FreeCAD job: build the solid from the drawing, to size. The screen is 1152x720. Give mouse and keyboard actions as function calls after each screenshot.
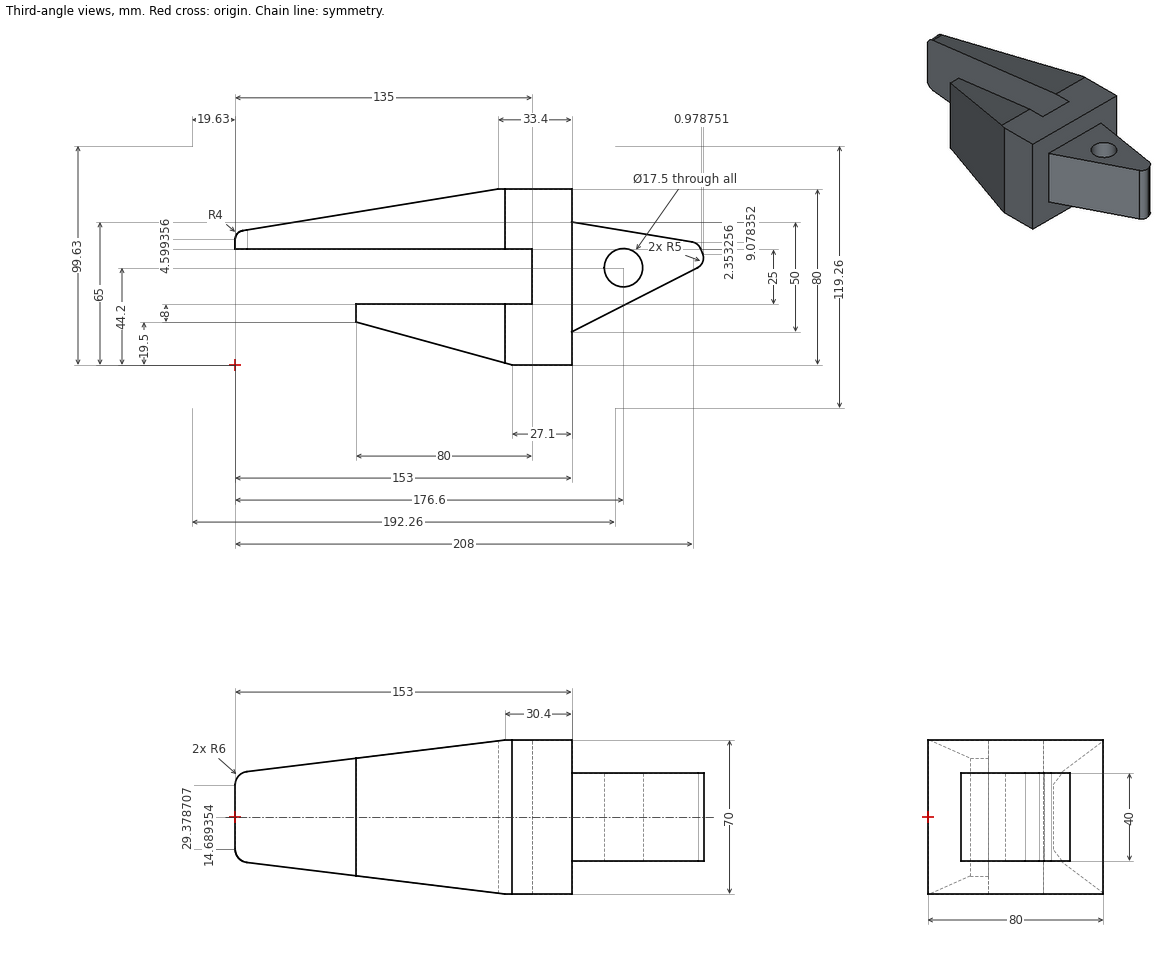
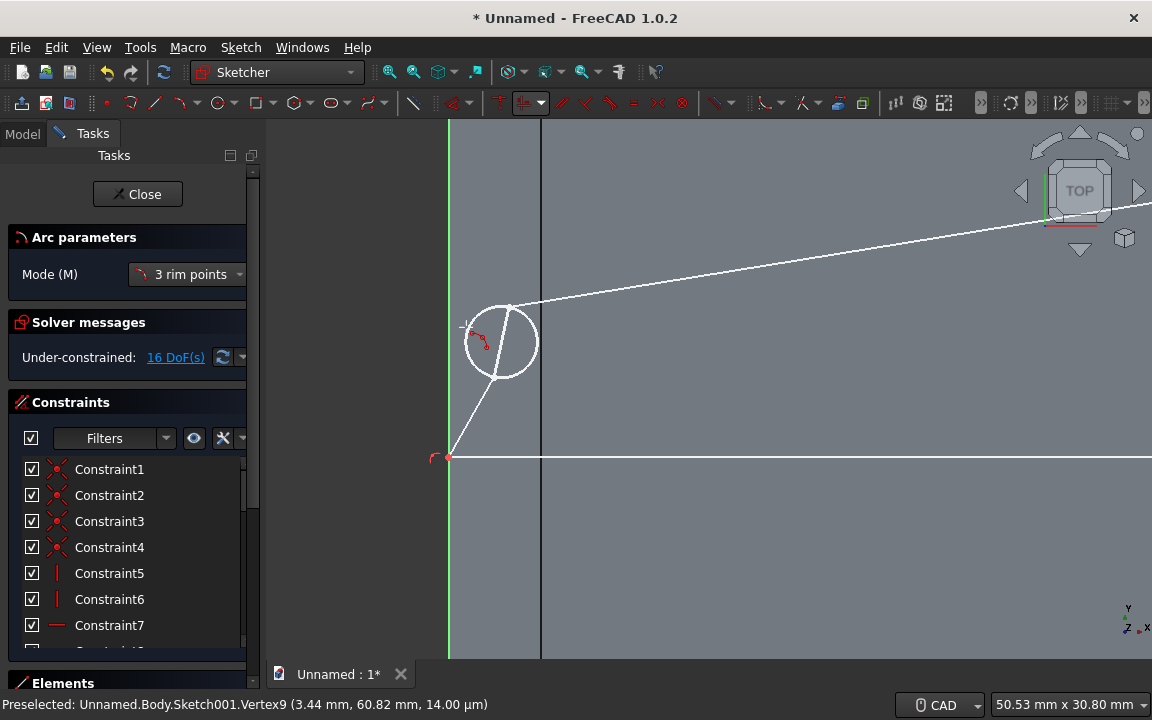
click(465, 327)
key(Escape)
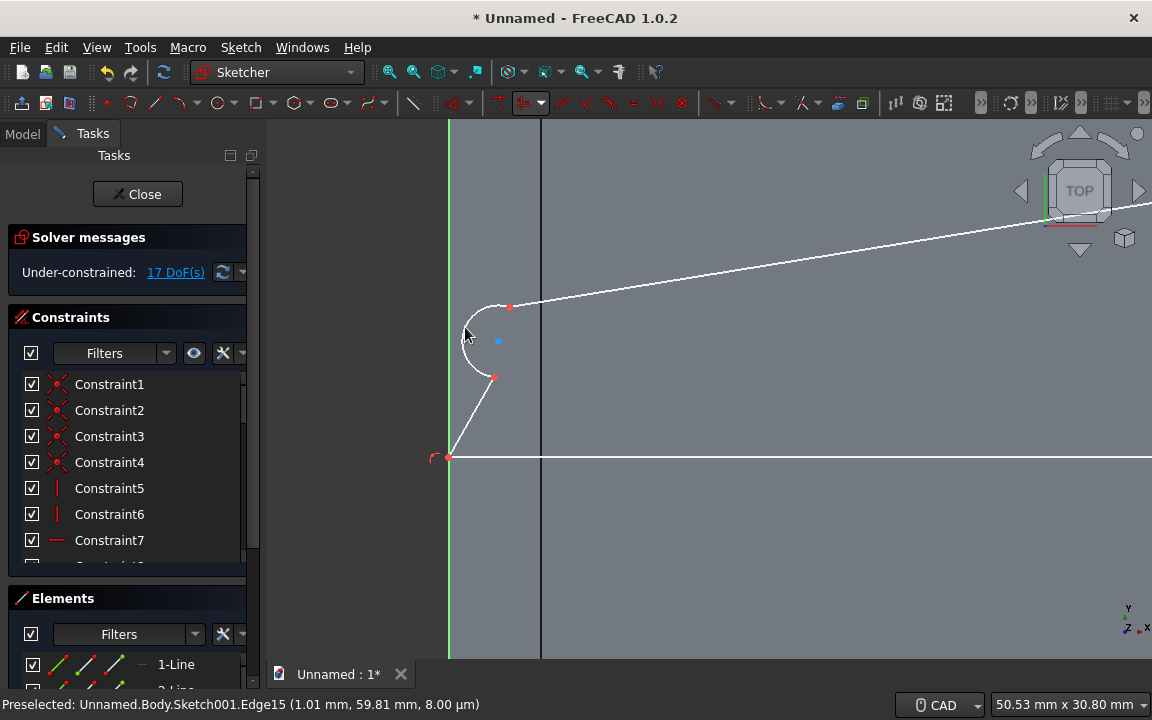
scroll(461, 345, down, 10)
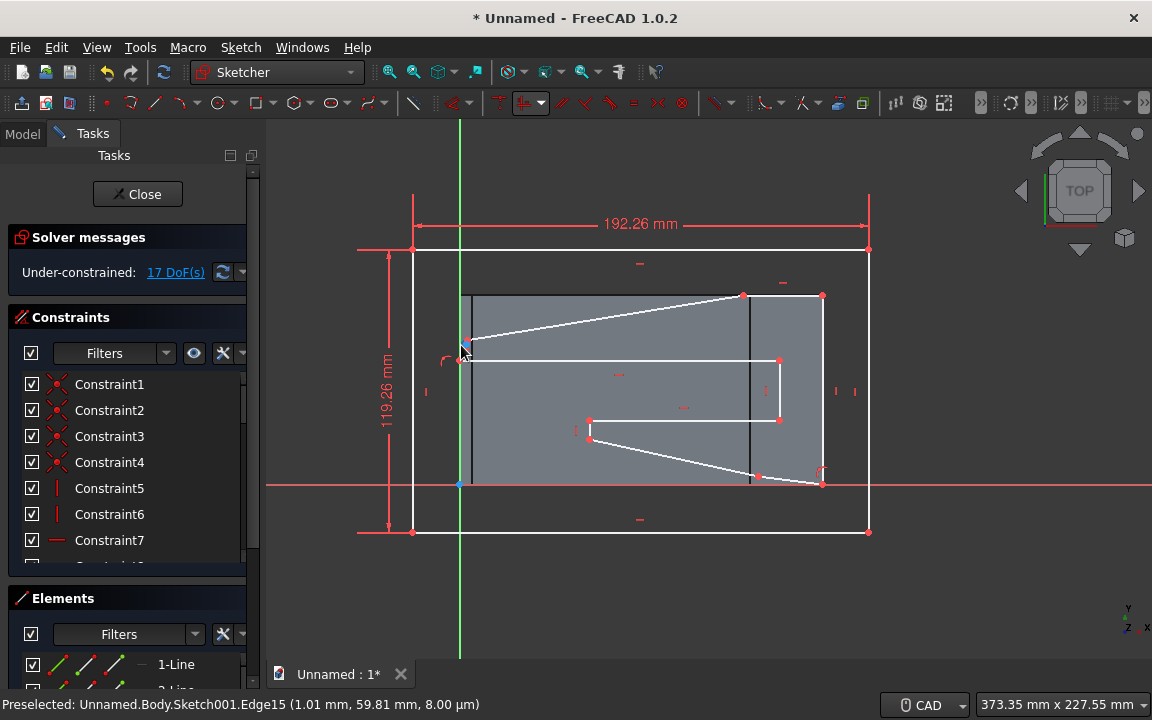
click(523, 331)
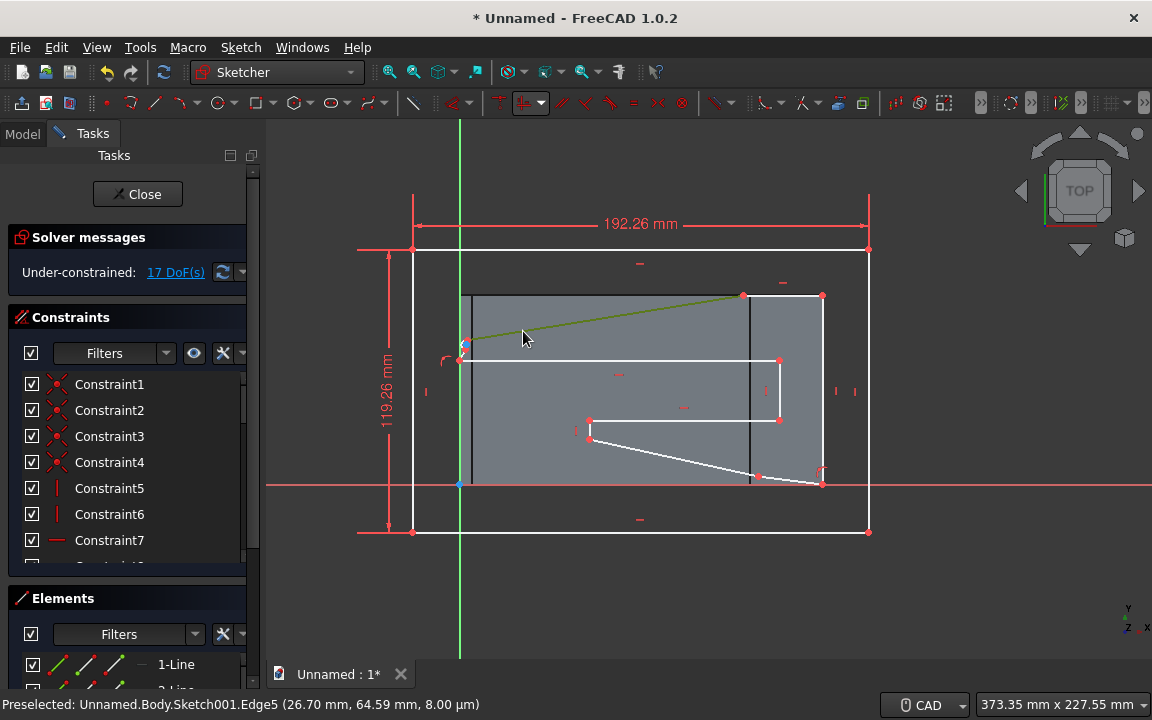
scroll(461, 344, up, 6)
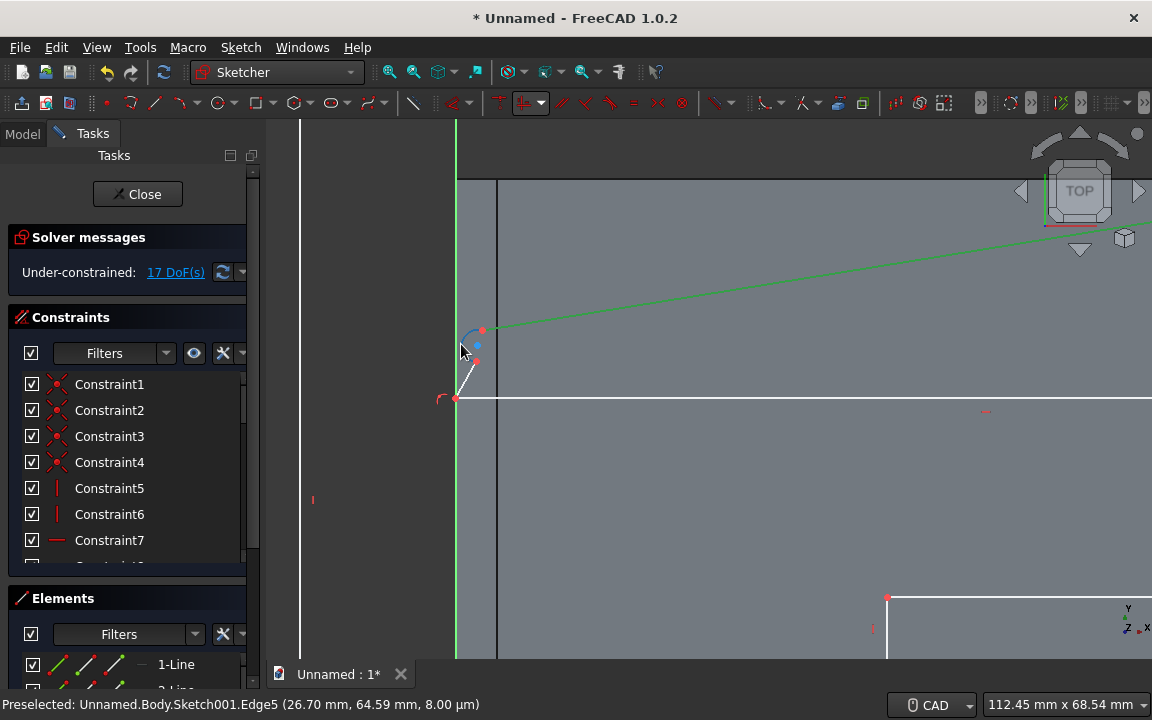
click(462, 343)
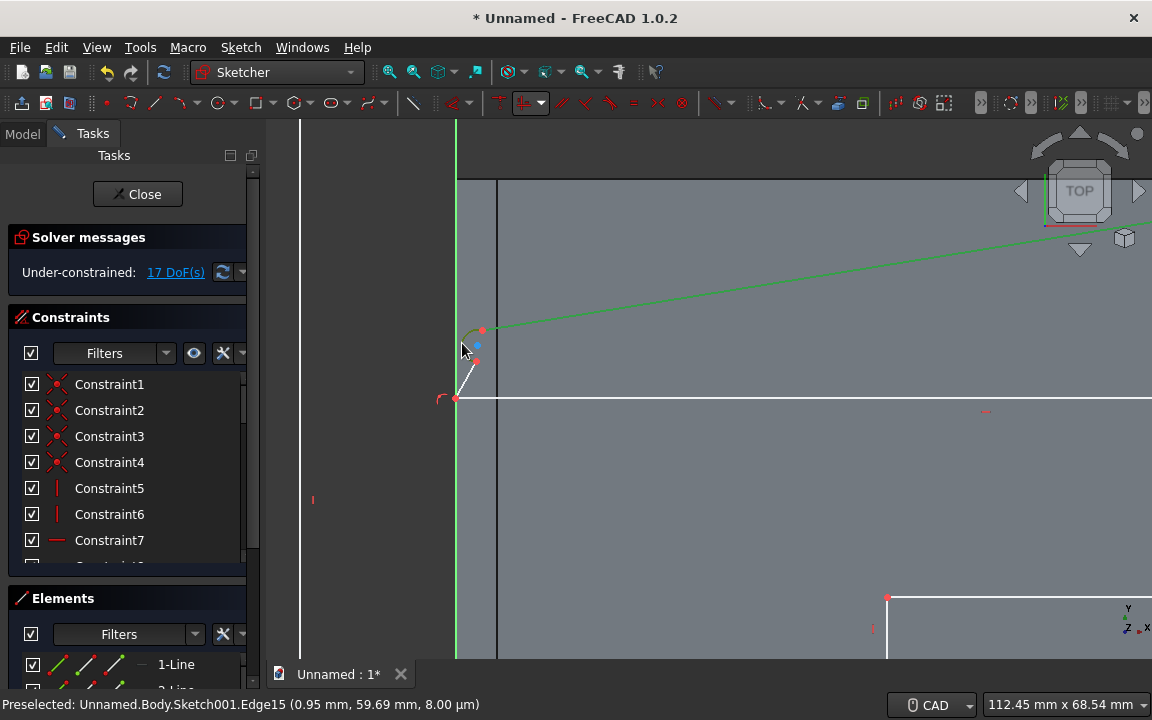
click(610, 104)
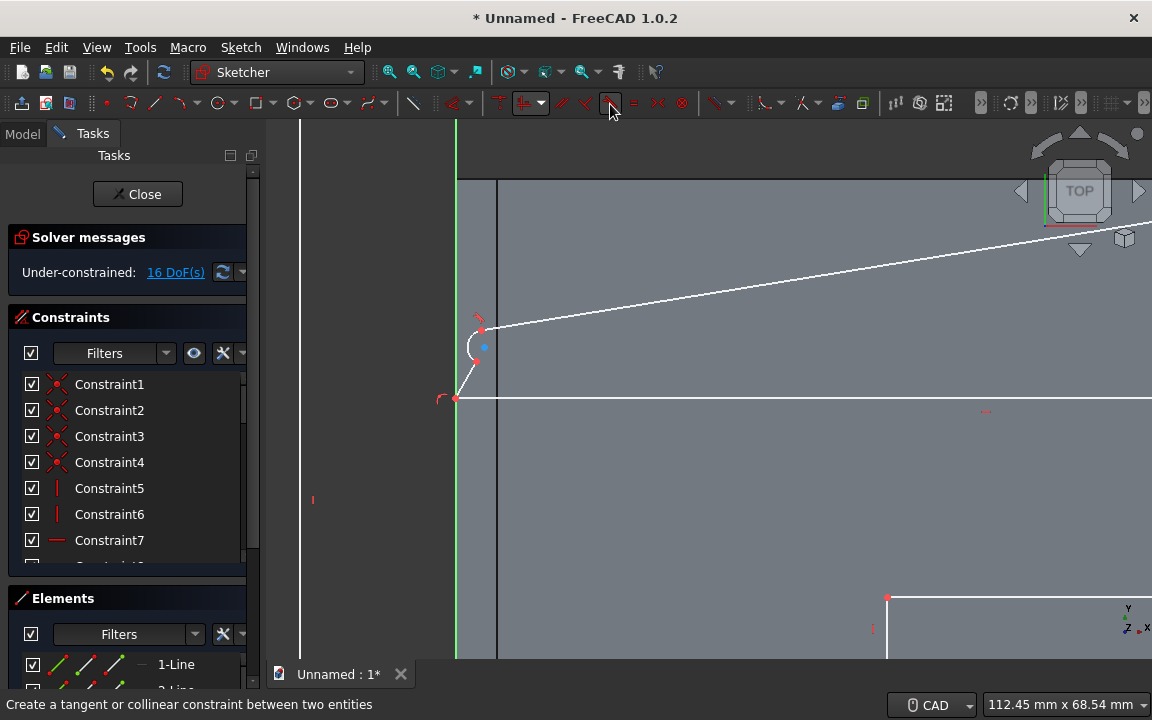
click(470, 373)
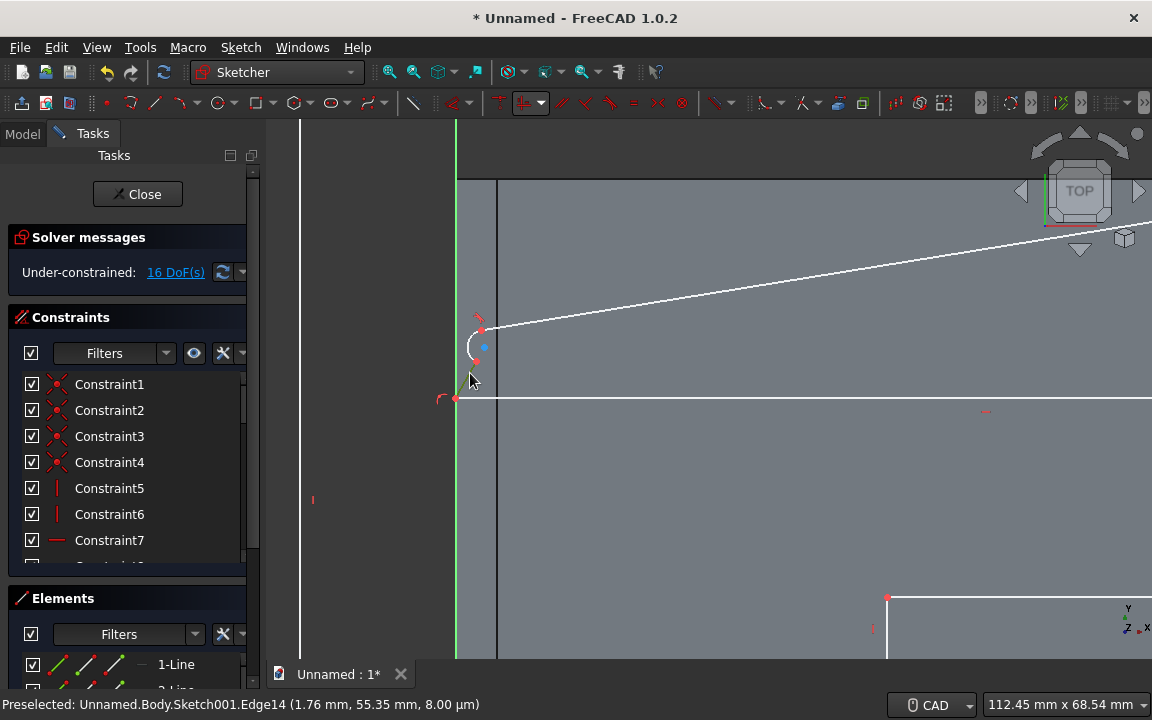
click(471, 337)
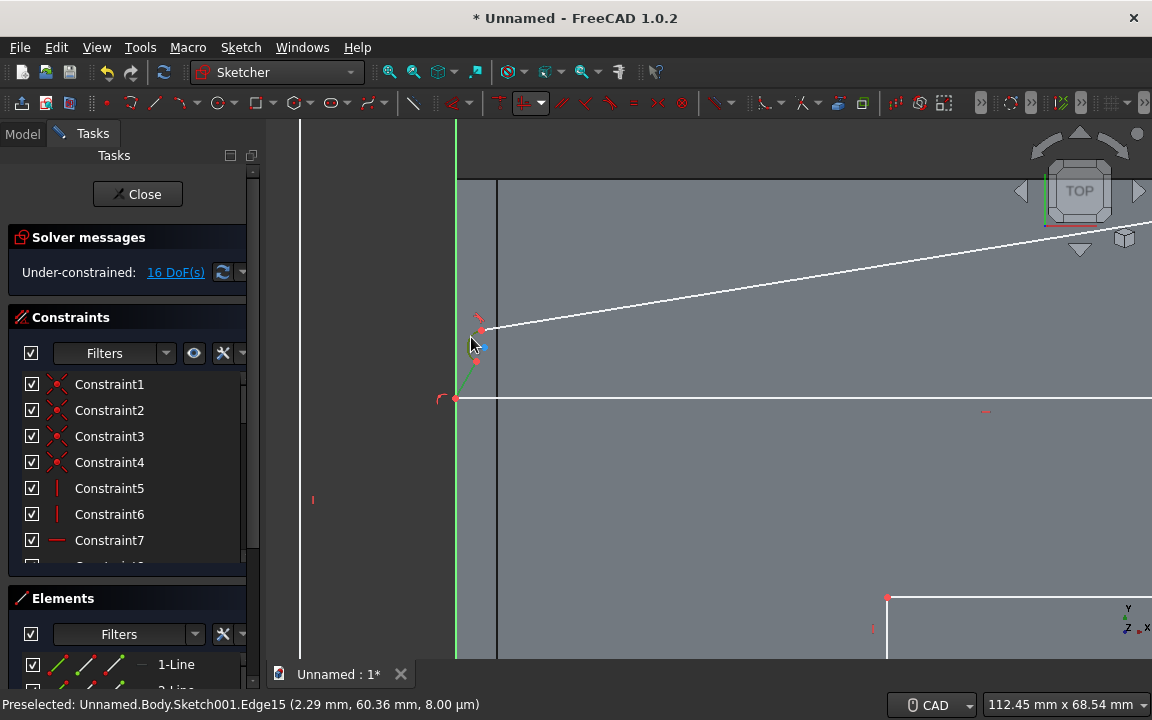
click(610, 104)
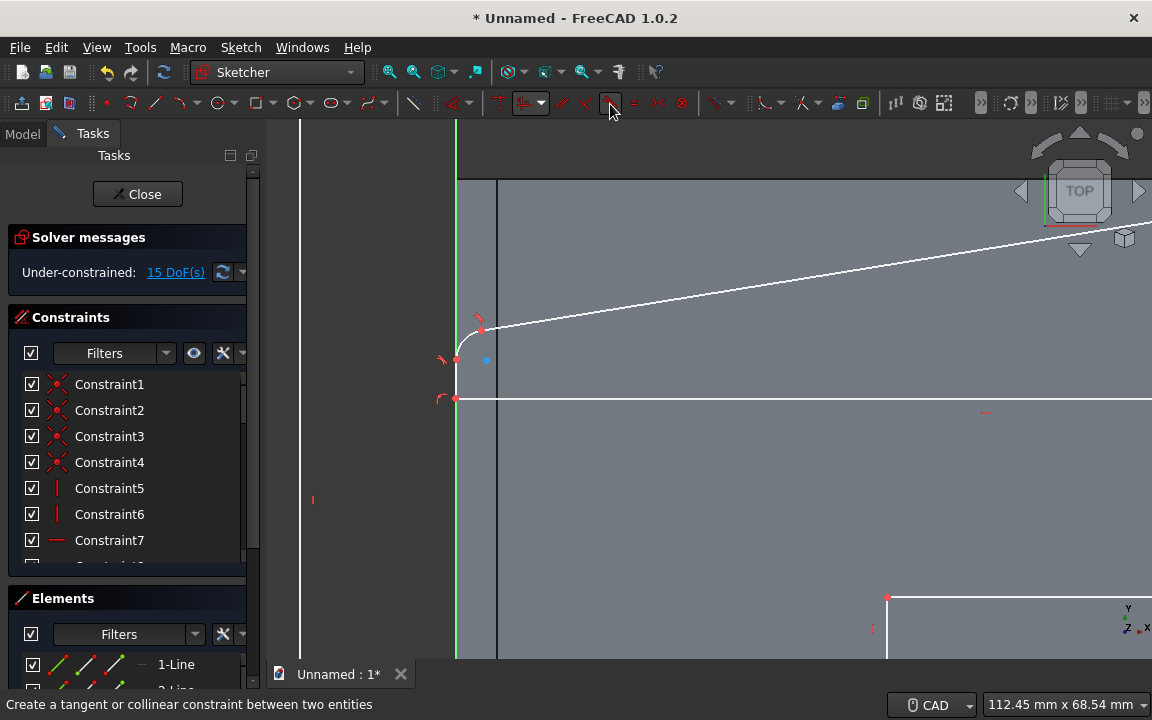
scroll(460, 343, down, 6)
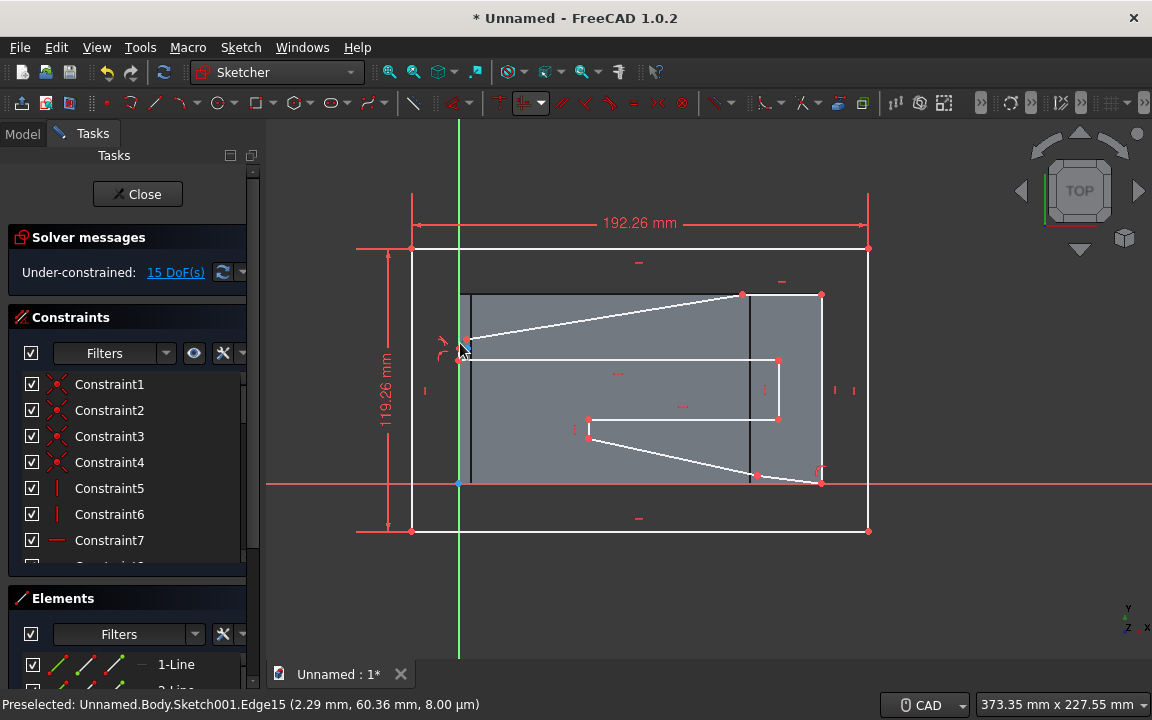
scroll(777, 478, up, 5)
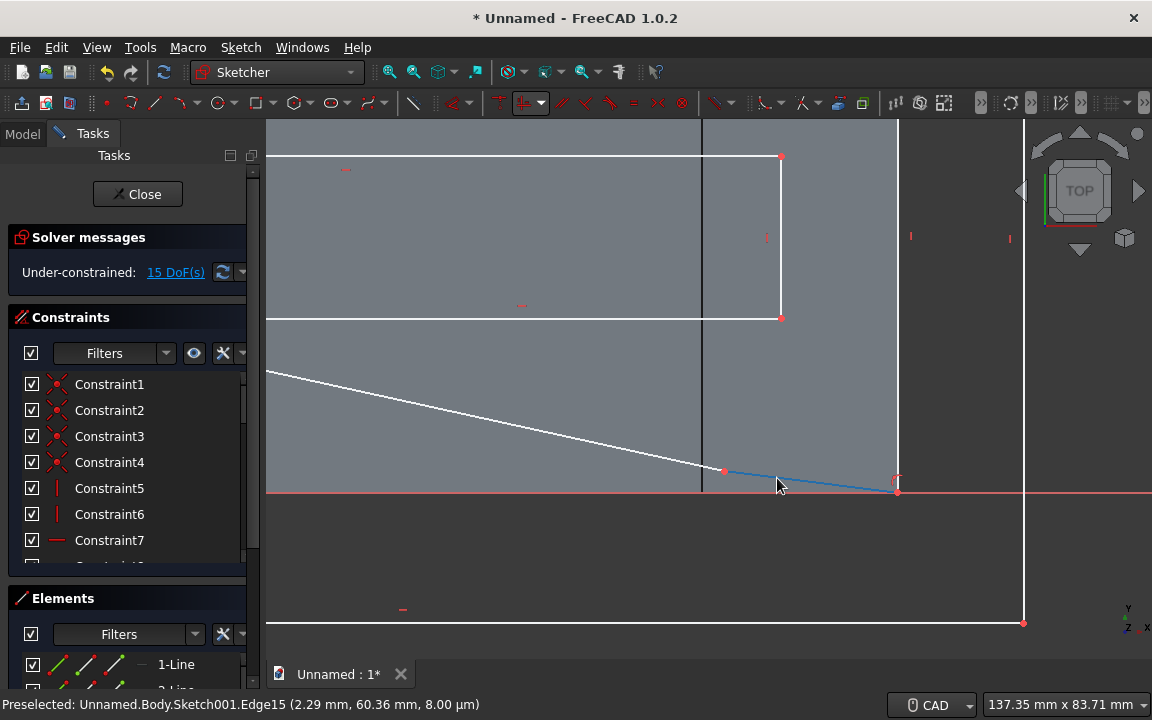
click(776, 478)